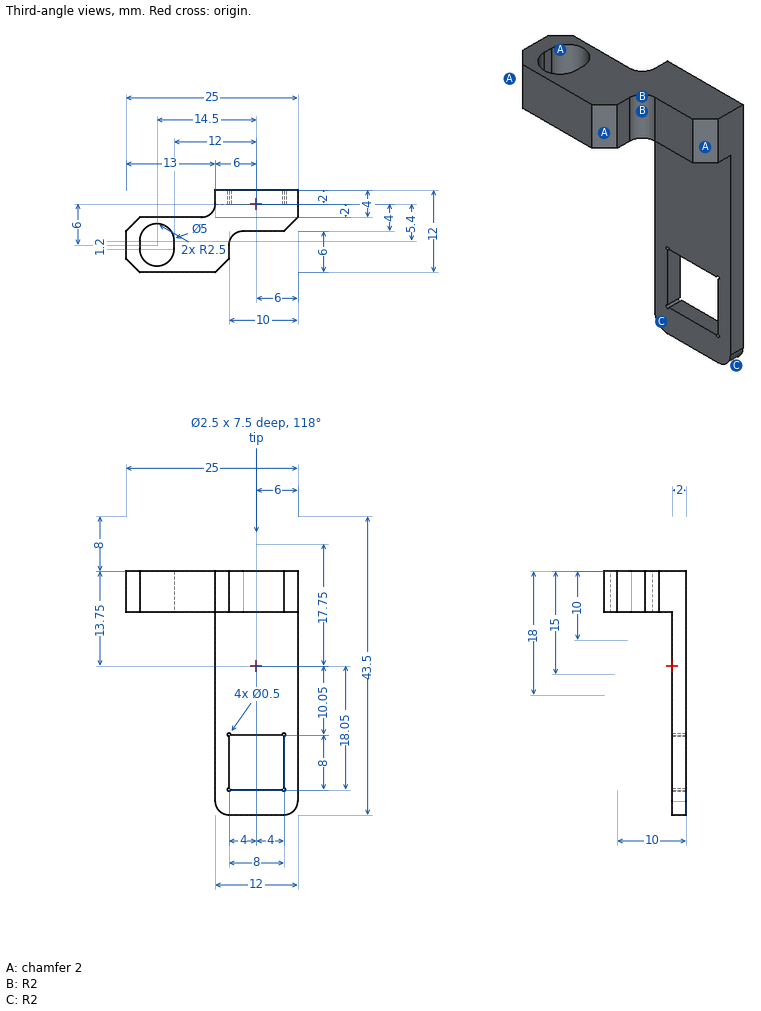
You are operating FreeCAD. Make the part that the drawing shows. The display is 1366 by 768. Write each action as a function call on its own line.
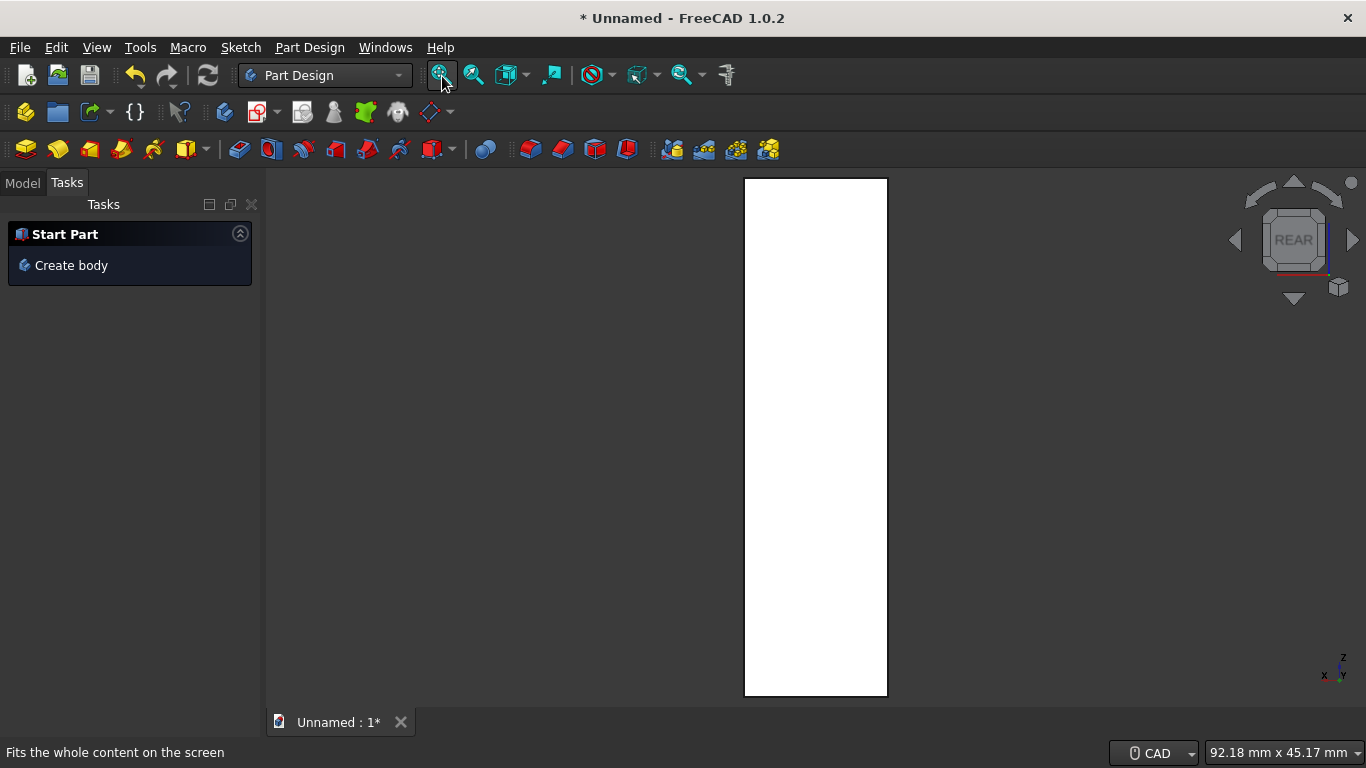
click(816, 288)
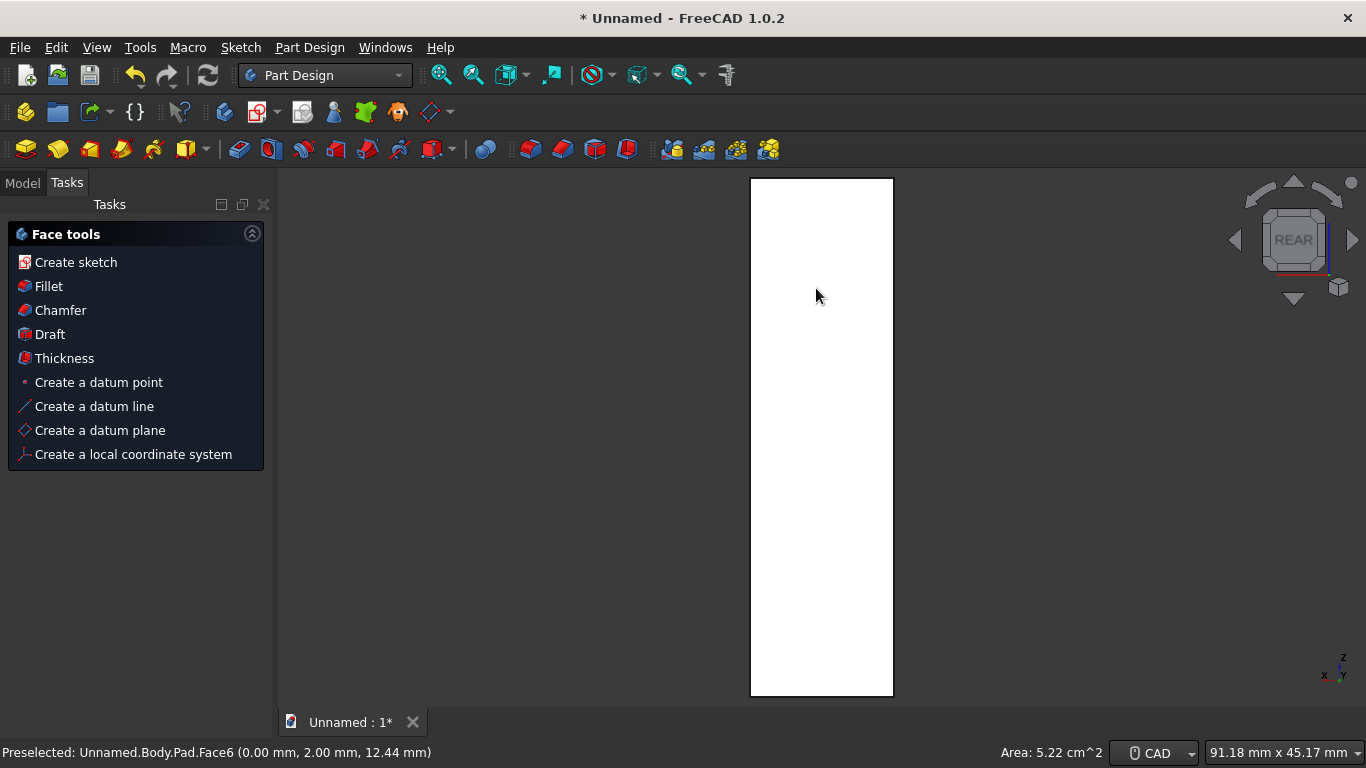
click(258, 112)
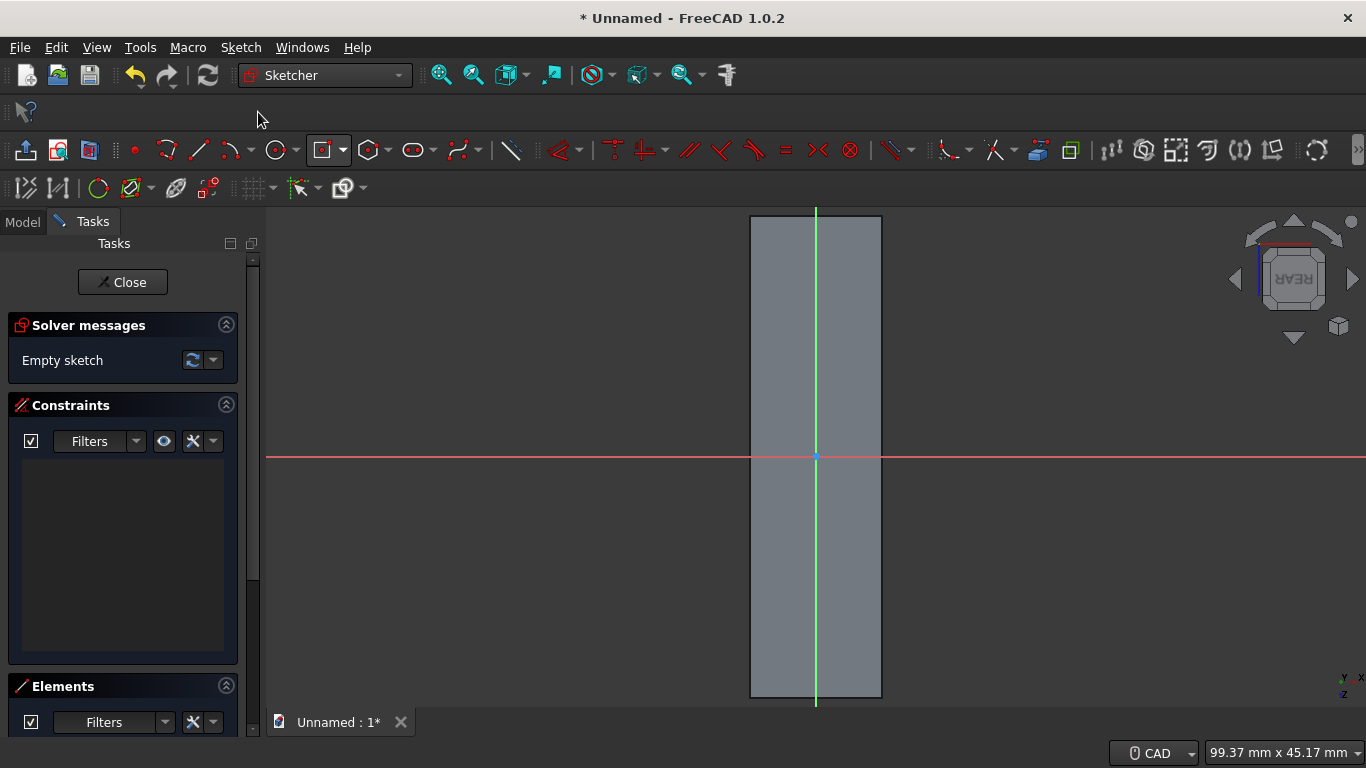
scroll(823, 673, up, 12)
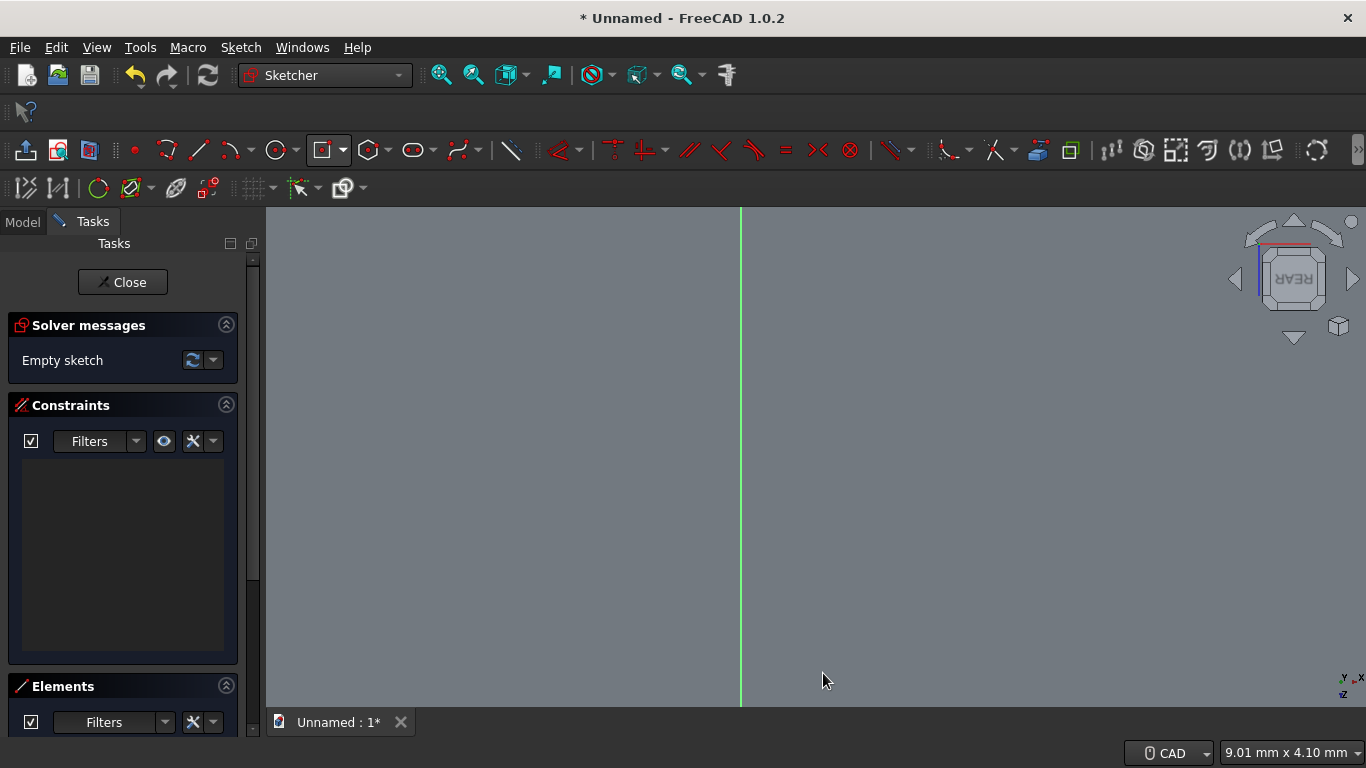
key(g)
key(c)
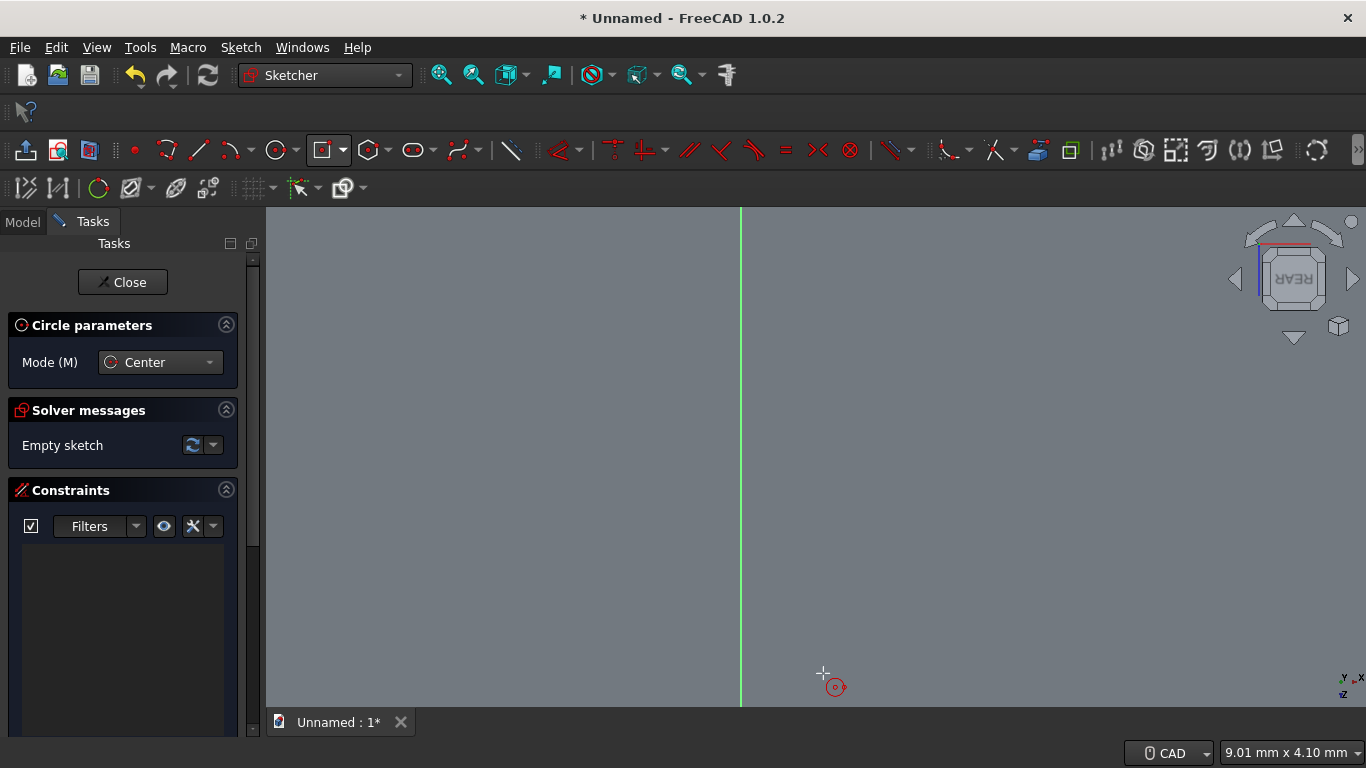
click(741, 449)
click(849, 341)
key(Escape)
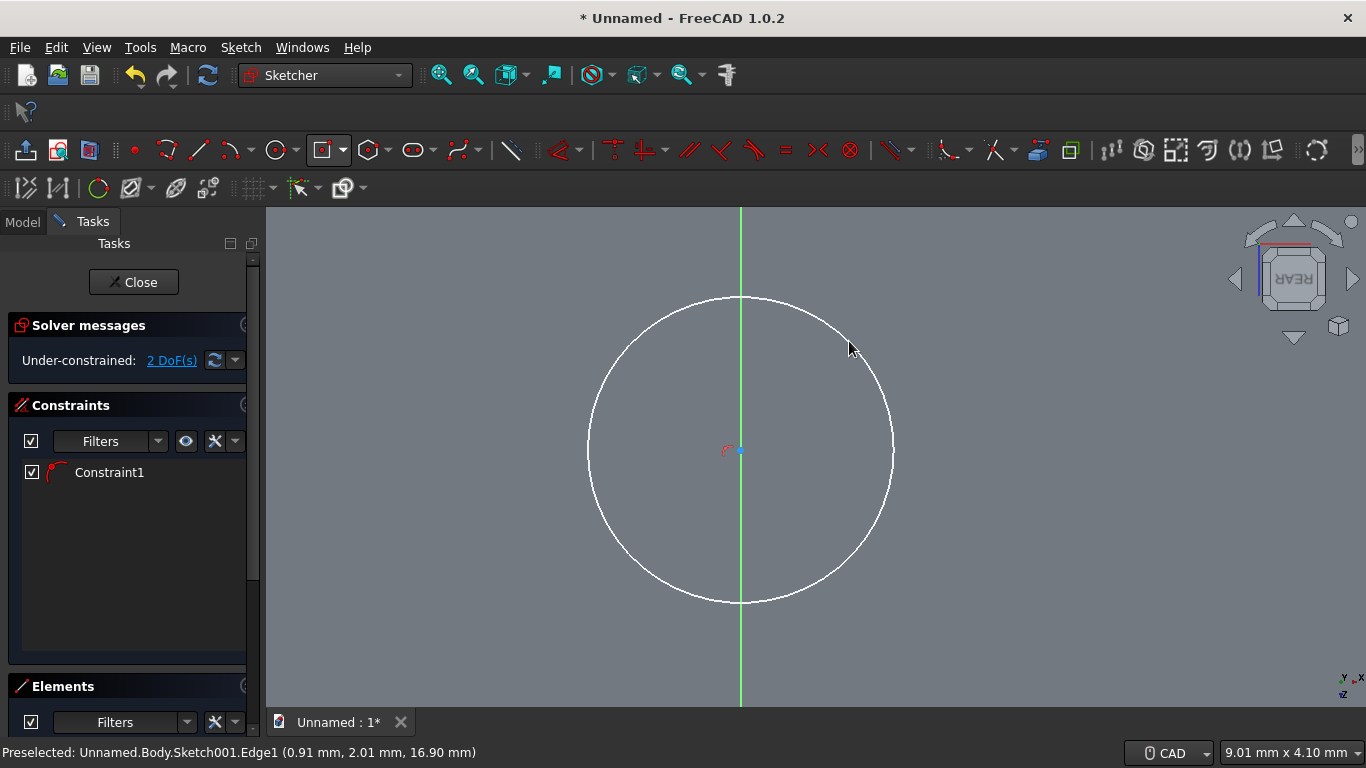
click(558, 150)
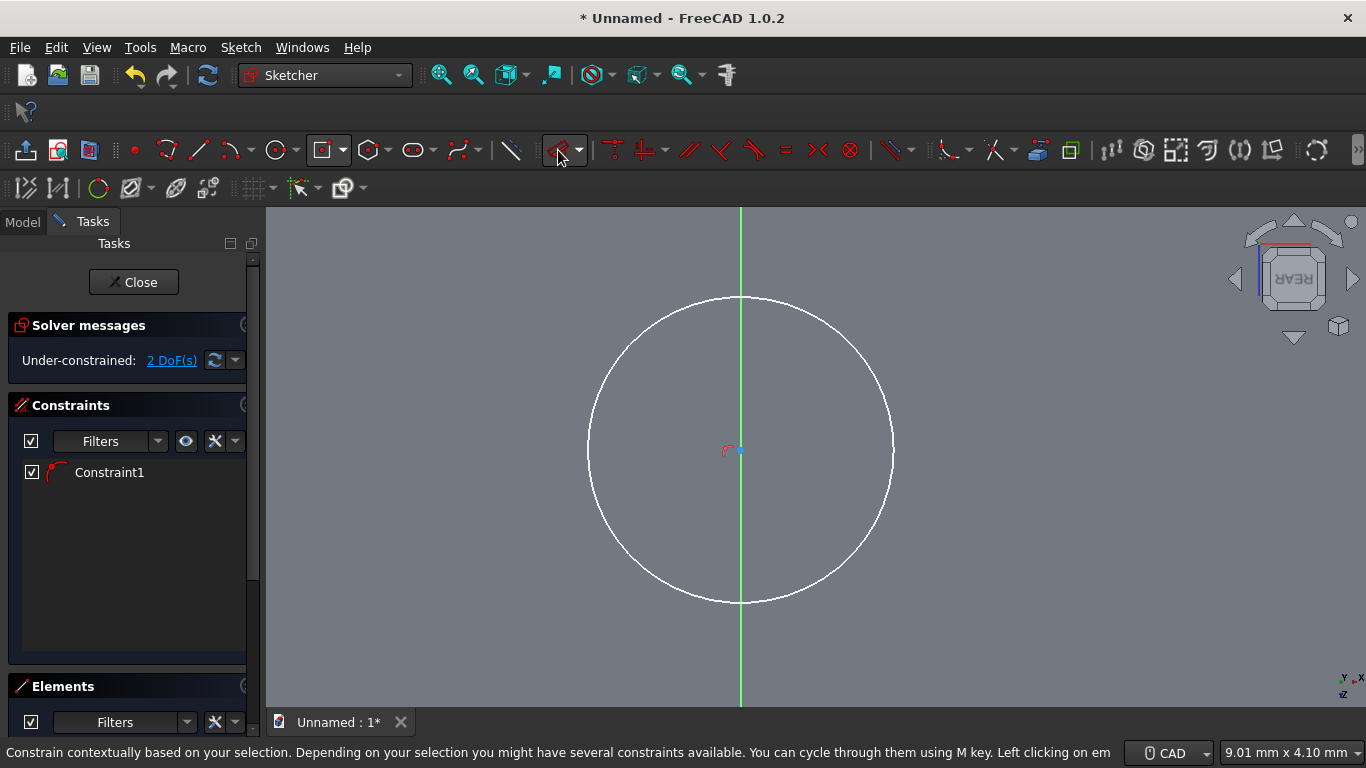
click(849, 342)
click(872, 319)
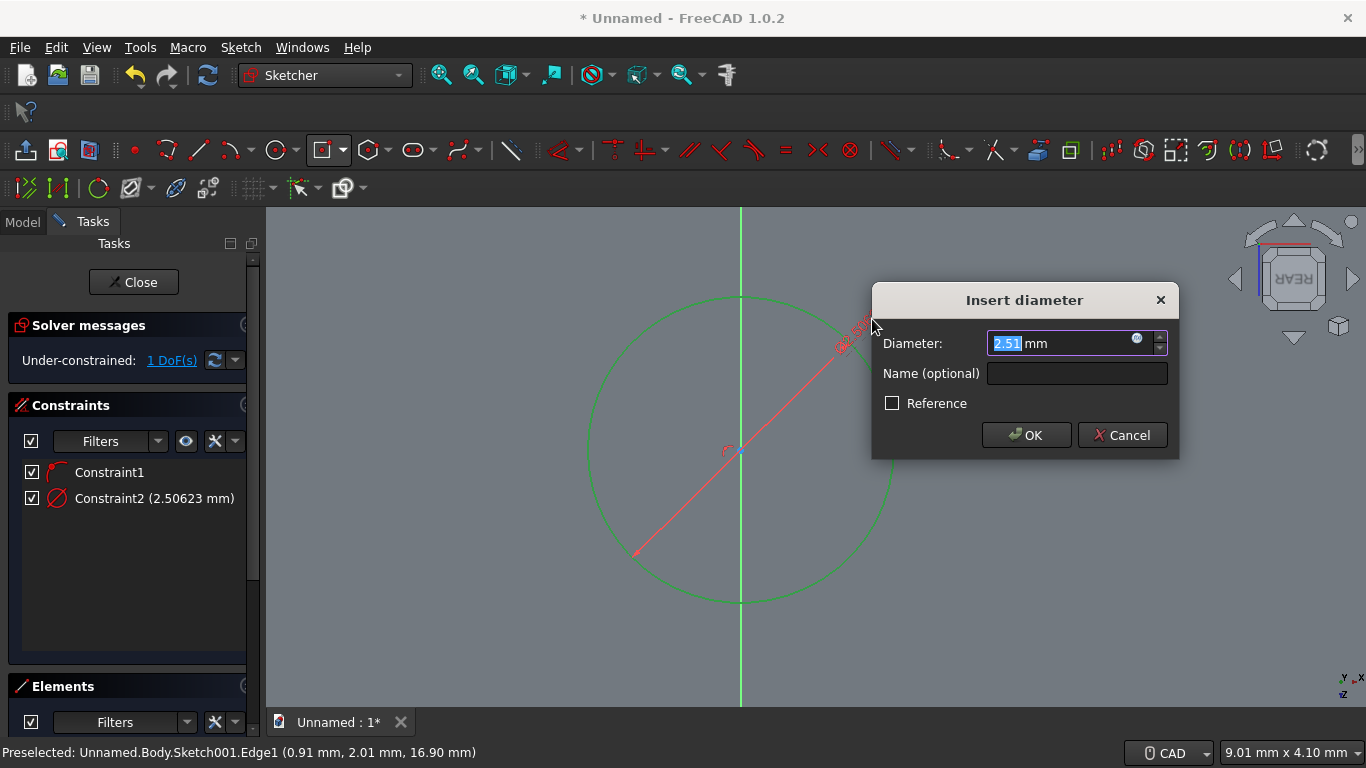
text(2.5)
key(Return)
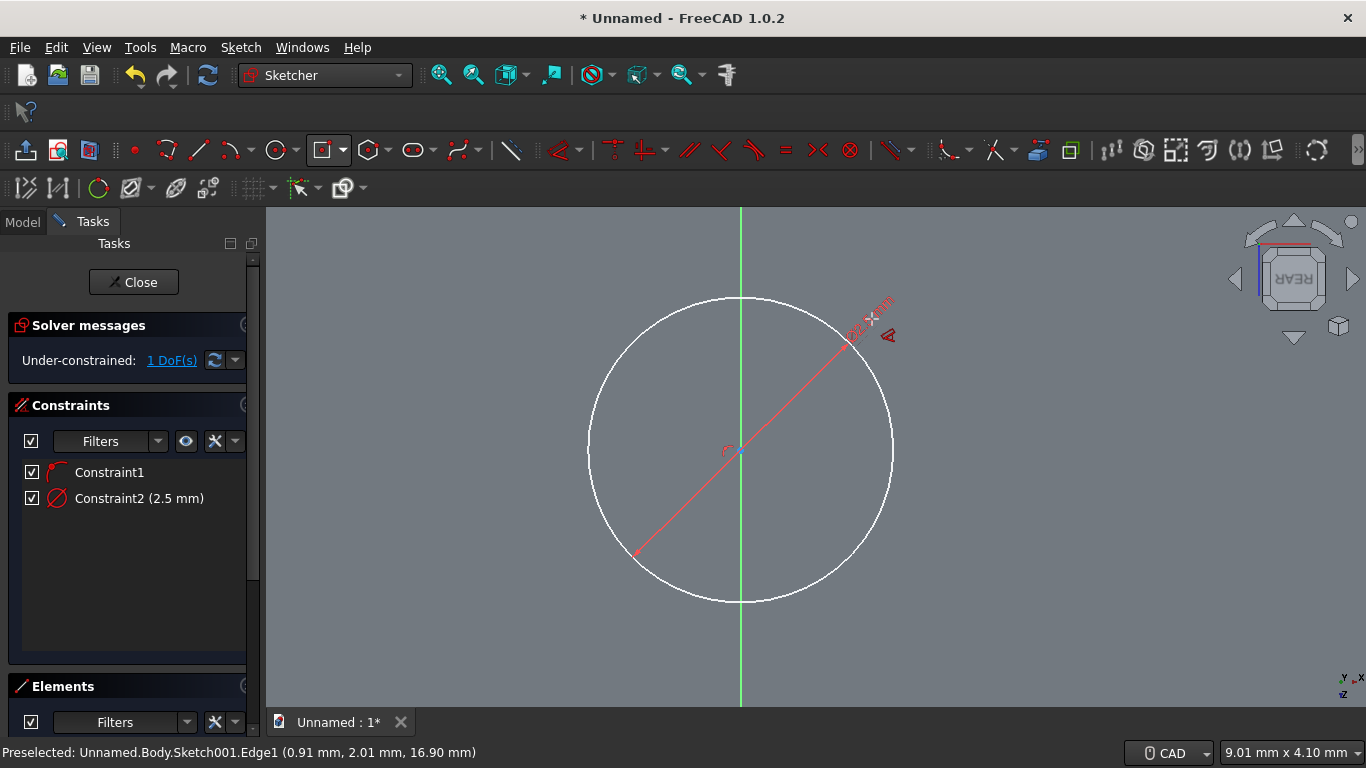
click(741, 450)
click(775, 342)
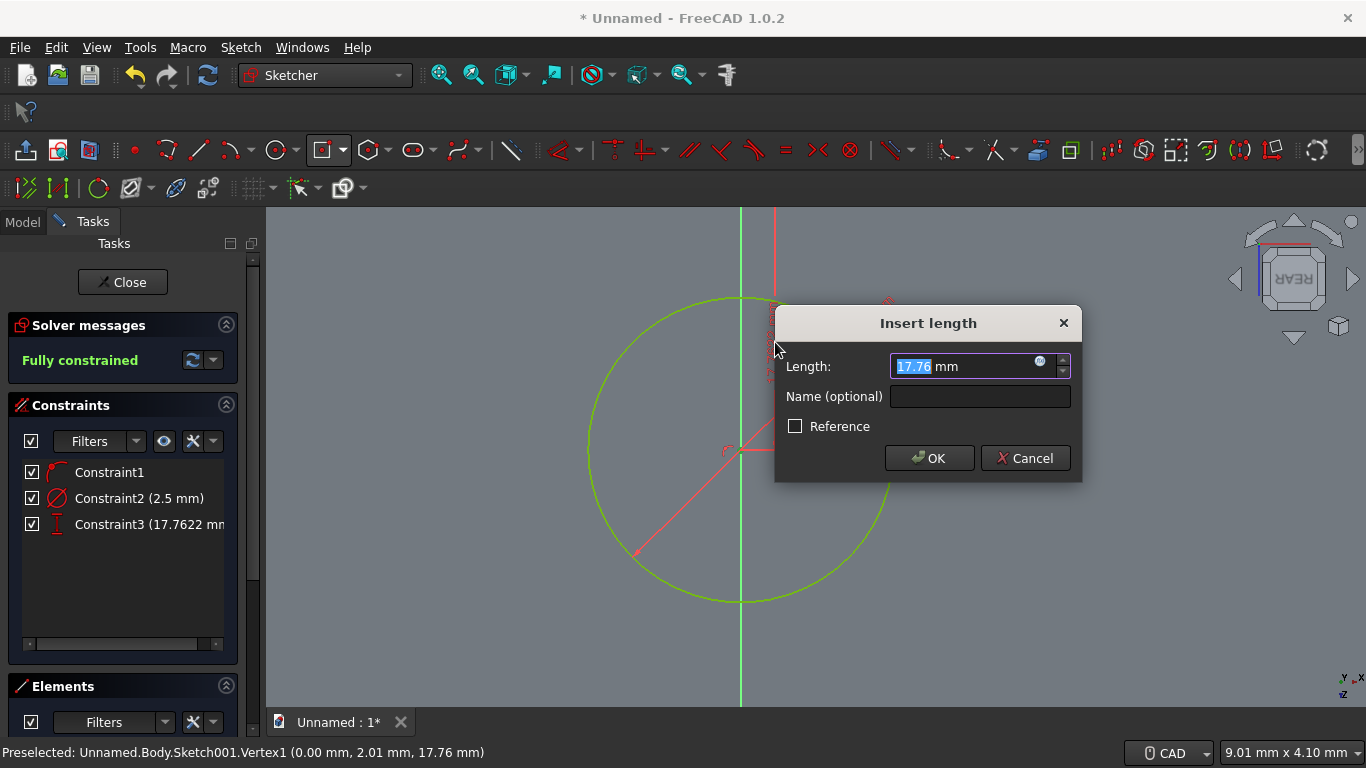
text(17.75)
key(Return)
key(Escape)